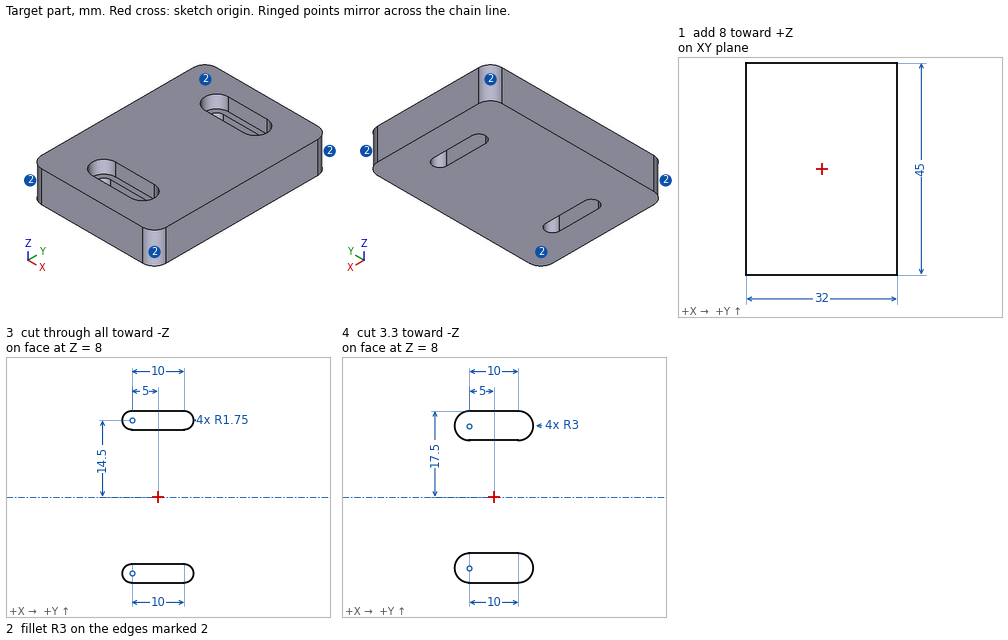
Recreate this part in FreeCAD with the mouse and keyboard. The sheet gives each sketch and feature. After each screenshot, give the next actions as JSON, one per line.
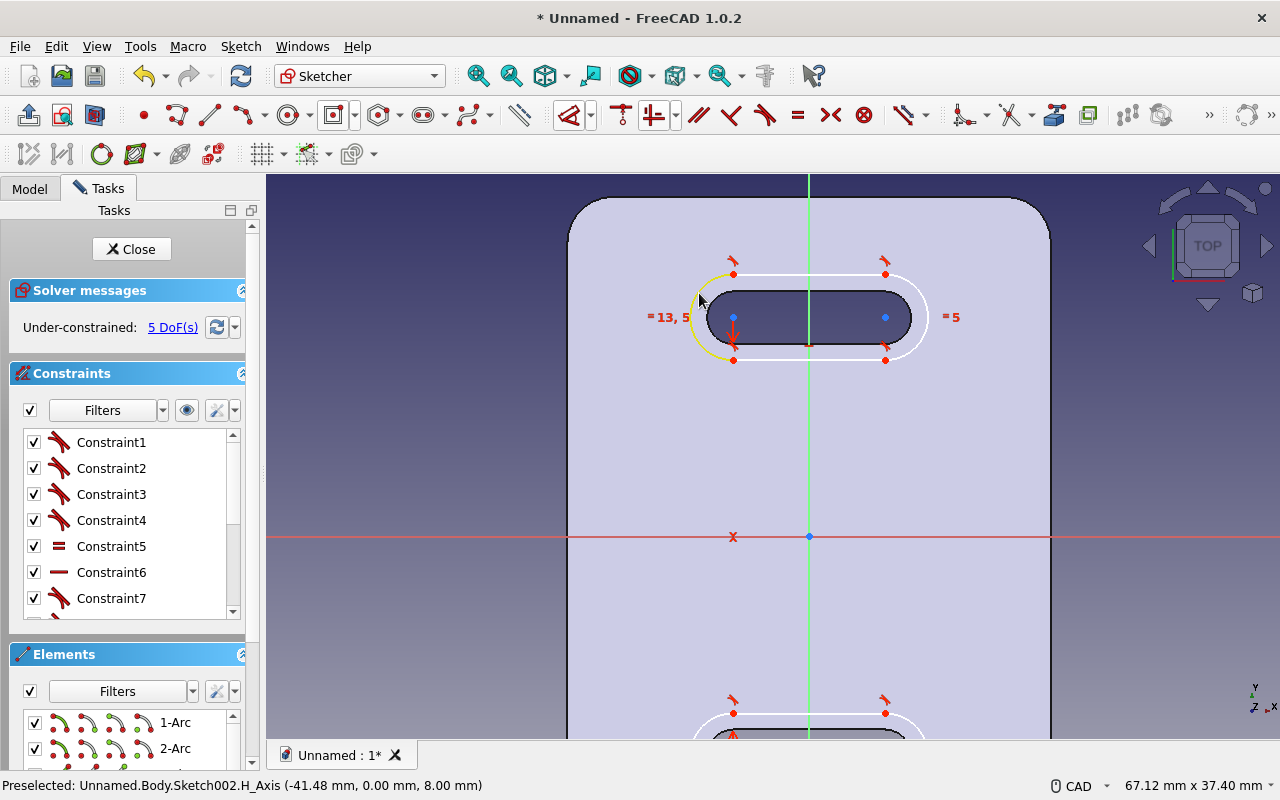
{"action": "left_click", "coordinate": [699, 292]}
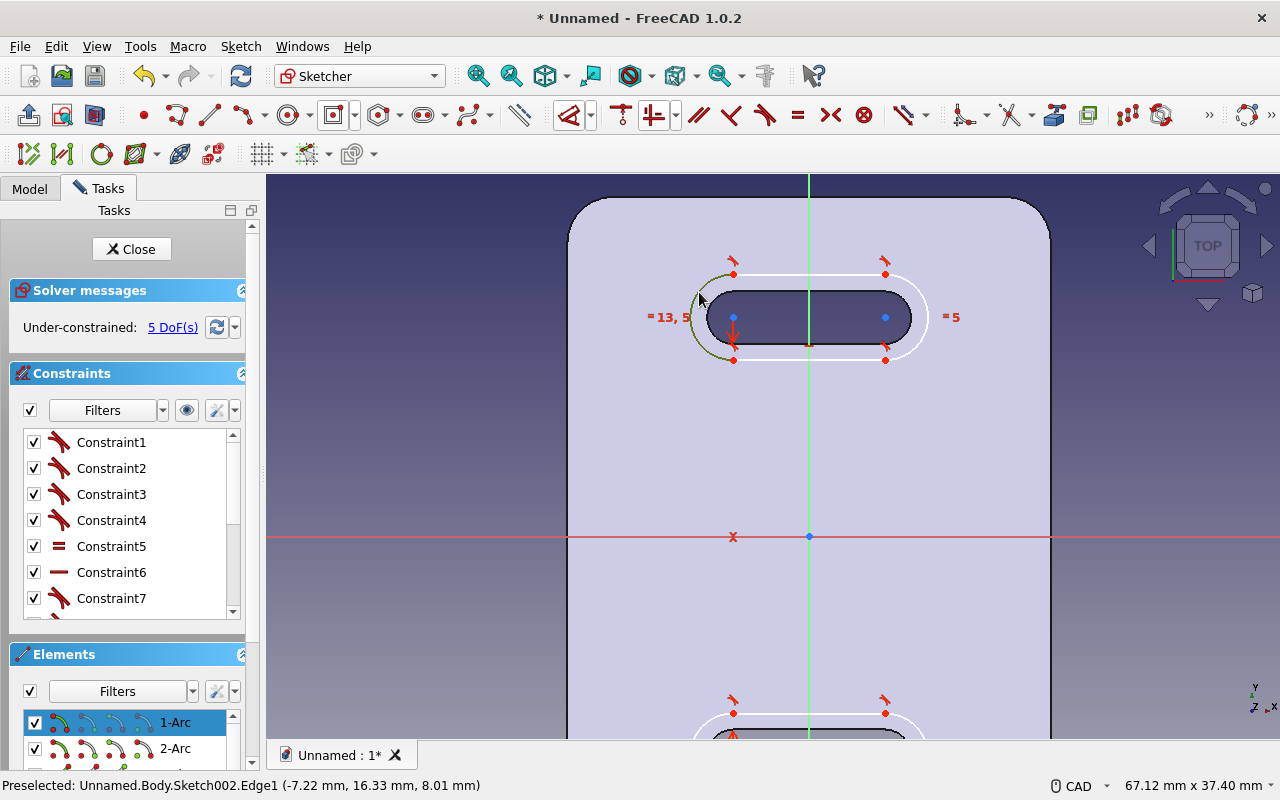
{"action": "key", "text": "k r"}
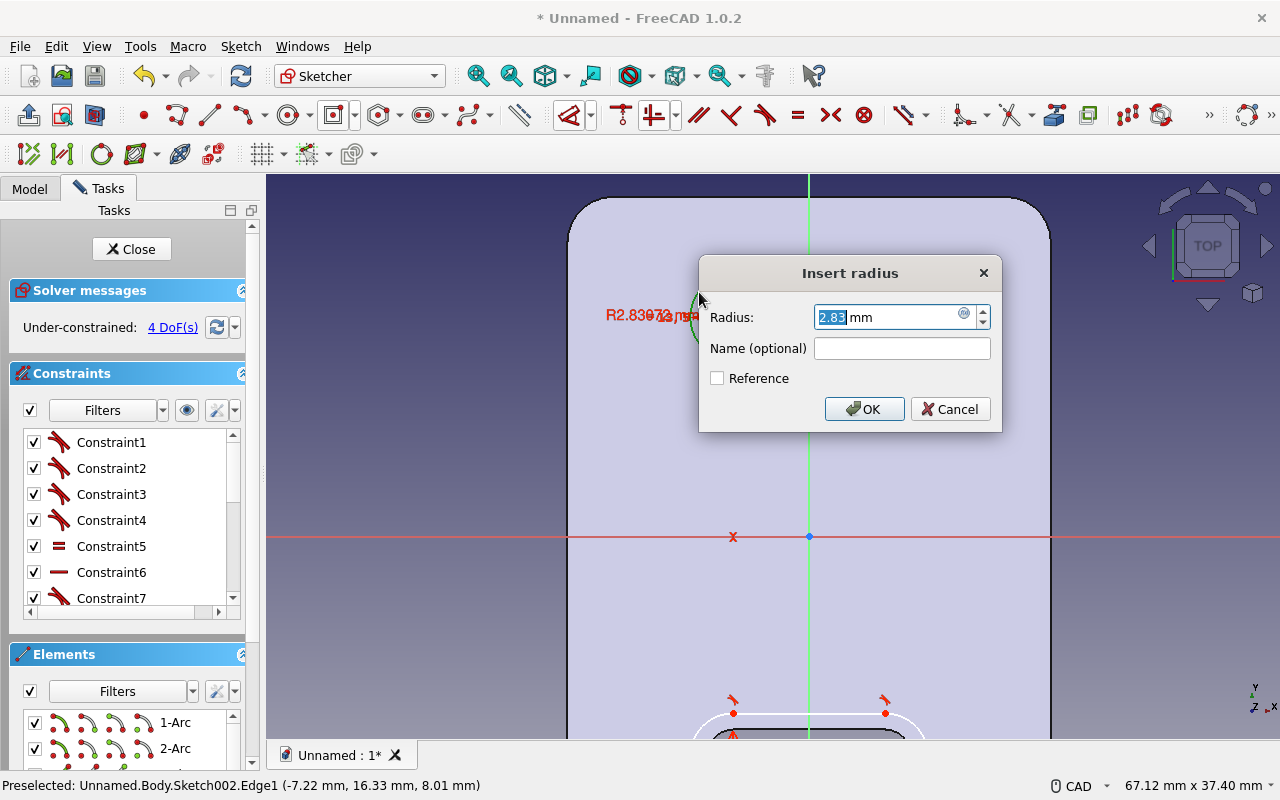
{"action": "type", "text": "3"}
{"action": "key", "text": "Return"}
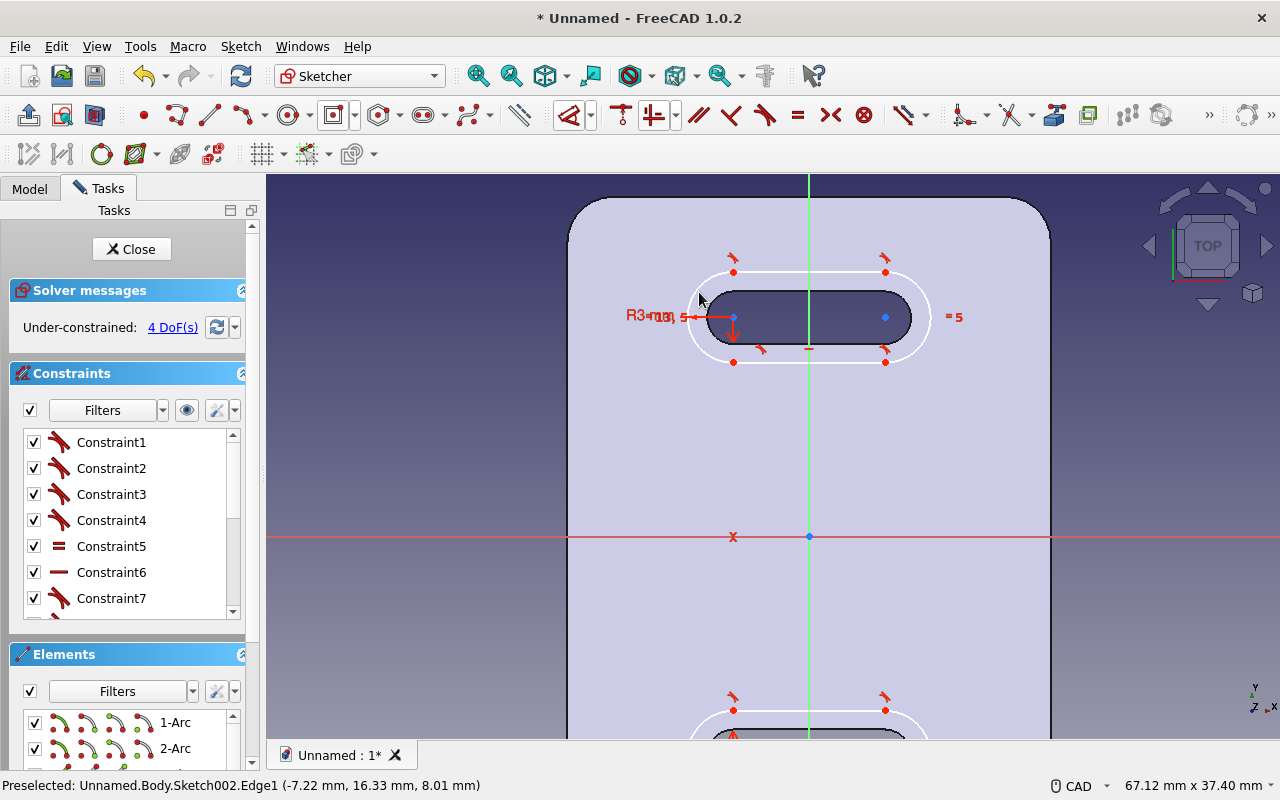
{"action": "left_click", "coordinate": [779, 272]}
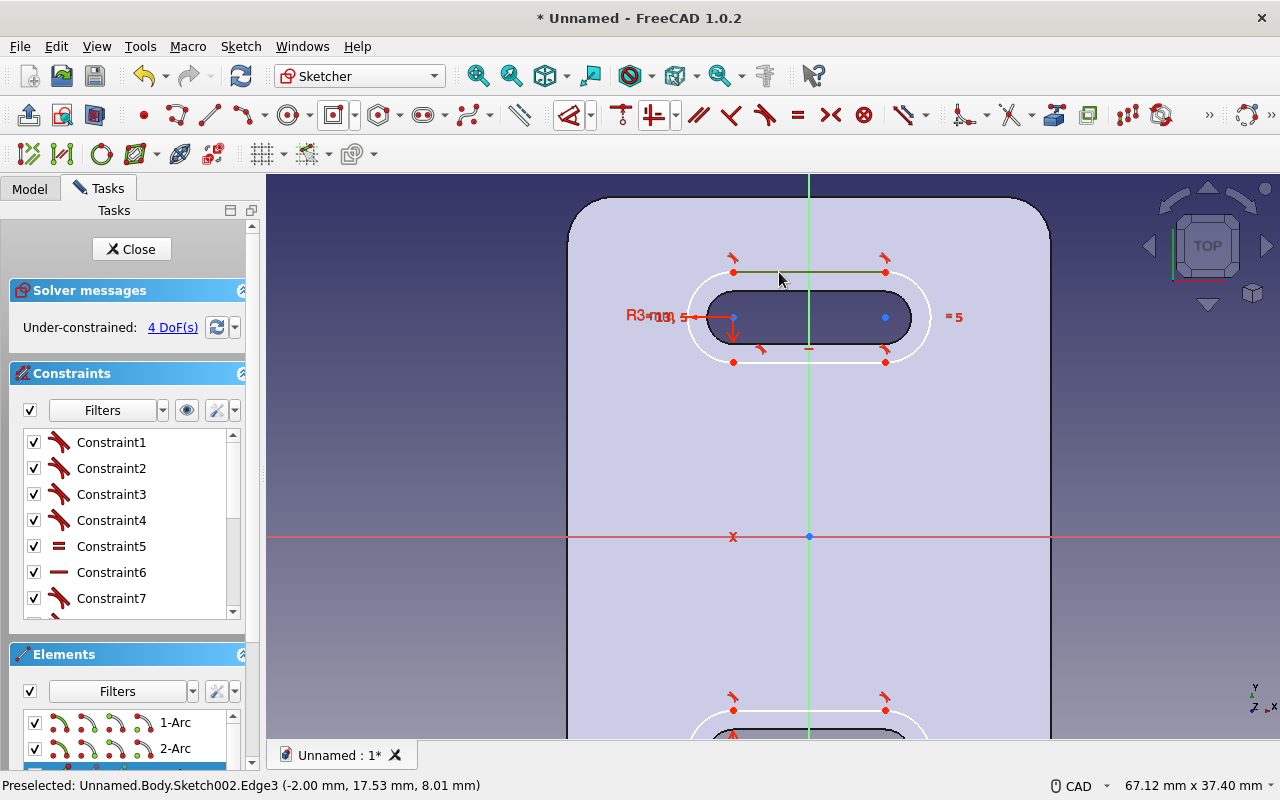
{"action": "key", "text": "l"}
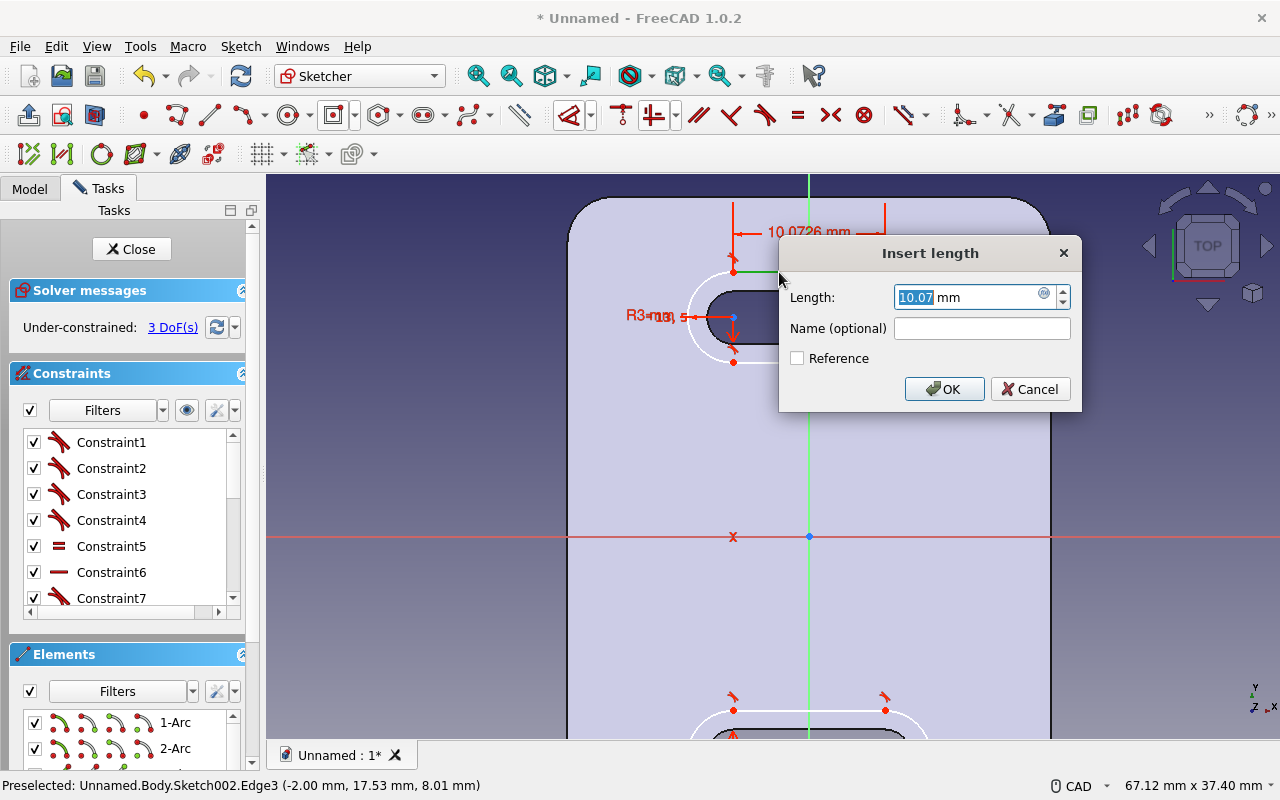
{"action": "type", "text": "10"}
{"action": "key", "text": "Return"}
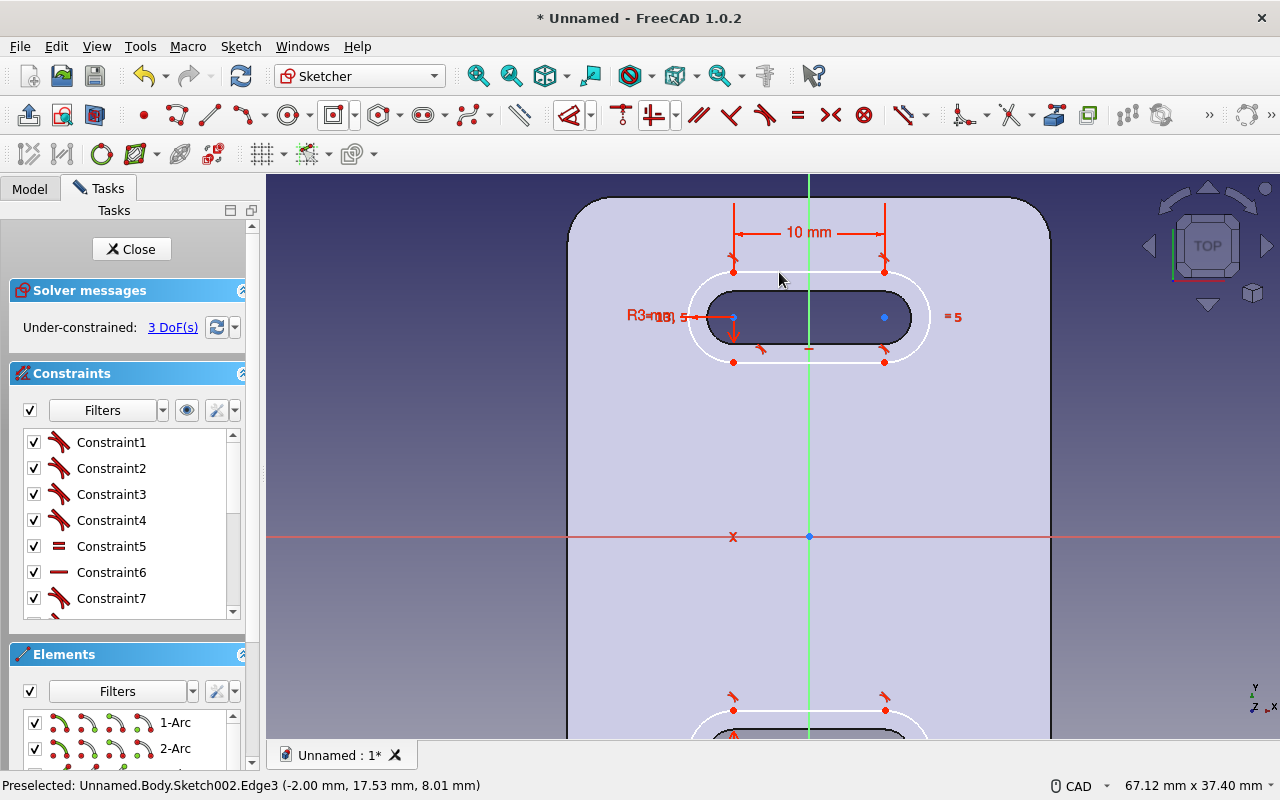
{"action": "left_click", "coordinate": [779, 711]}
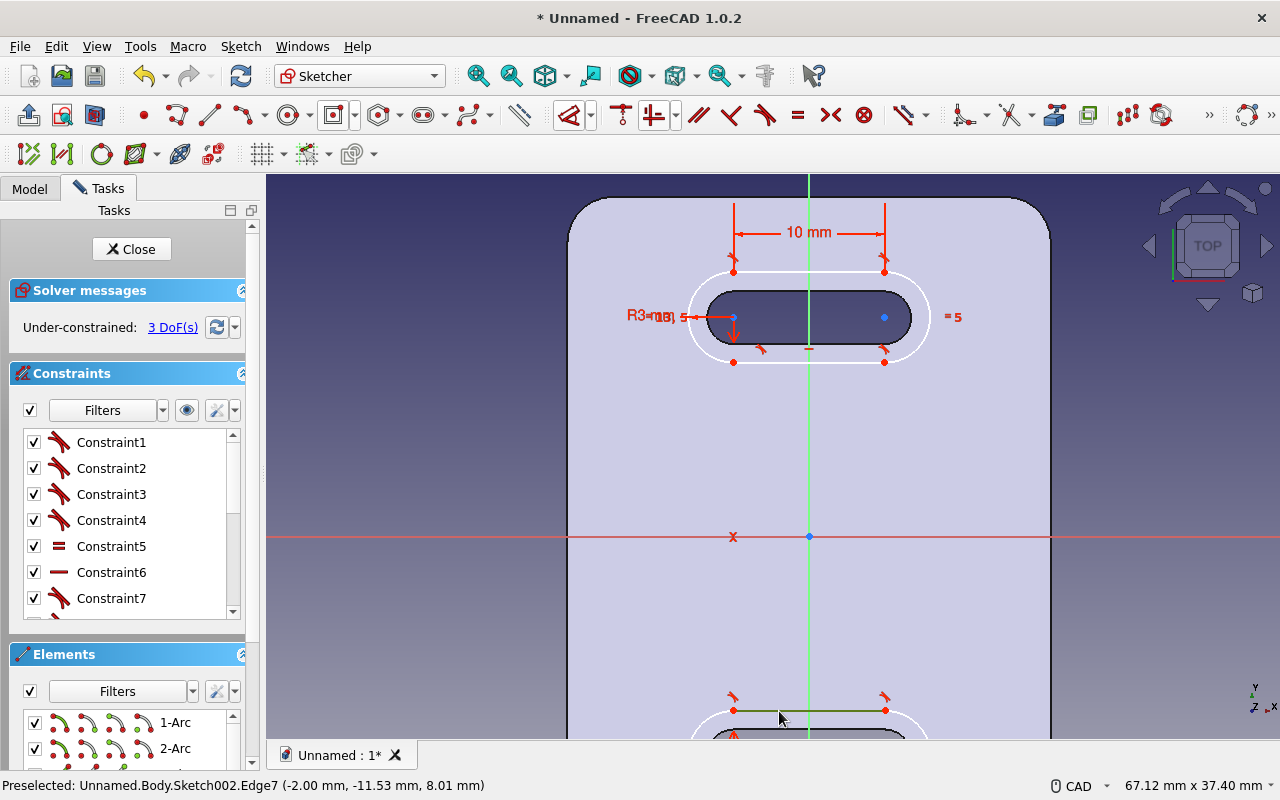
{"action": "left_click", "coordinate": [590, 116]}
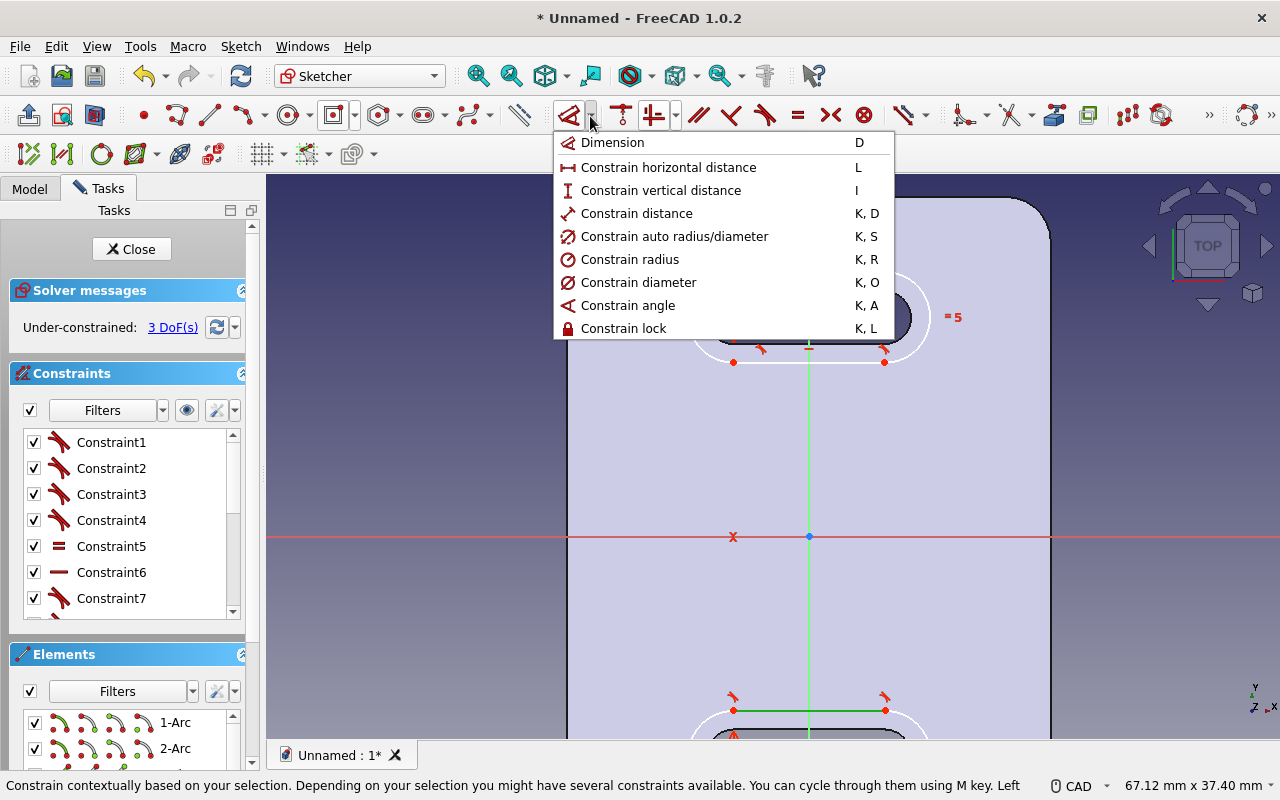
{"action": "left_click", "coordinate": [724, 168]}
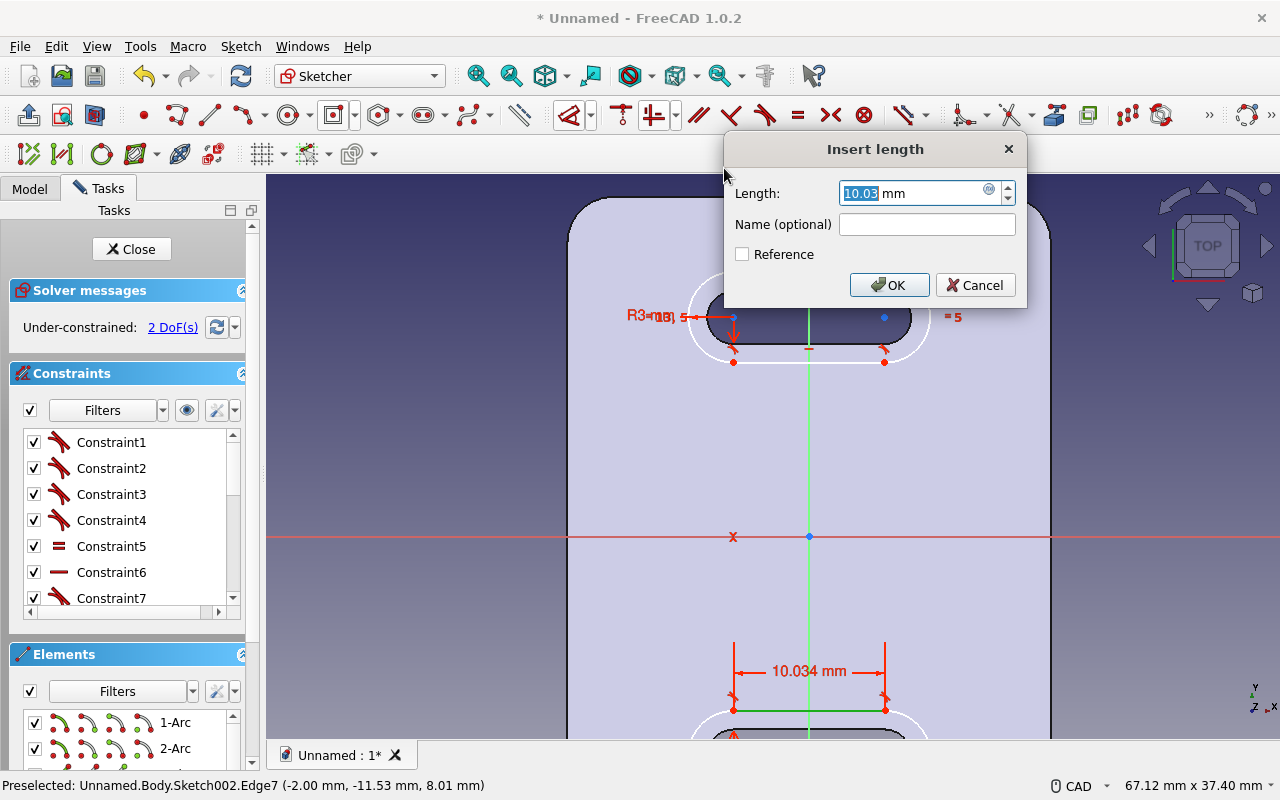
{"action": "type", "text": "10"}
{"action": "key", "text": "Return"}